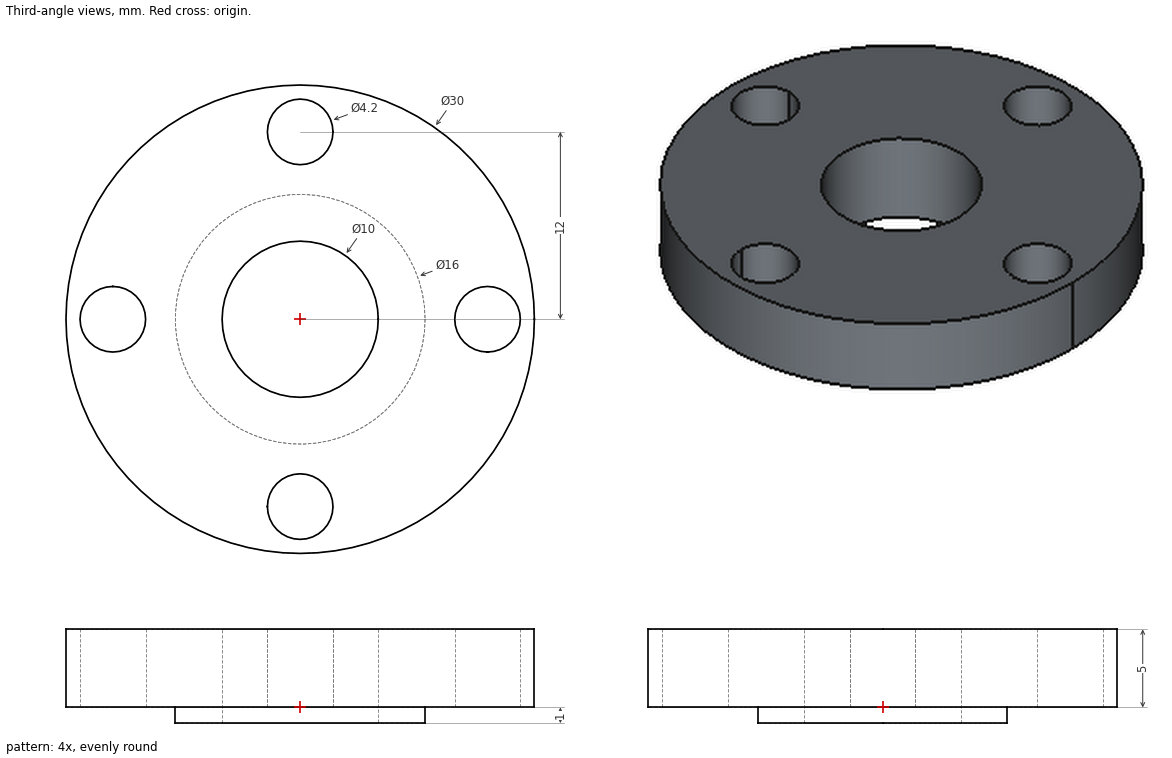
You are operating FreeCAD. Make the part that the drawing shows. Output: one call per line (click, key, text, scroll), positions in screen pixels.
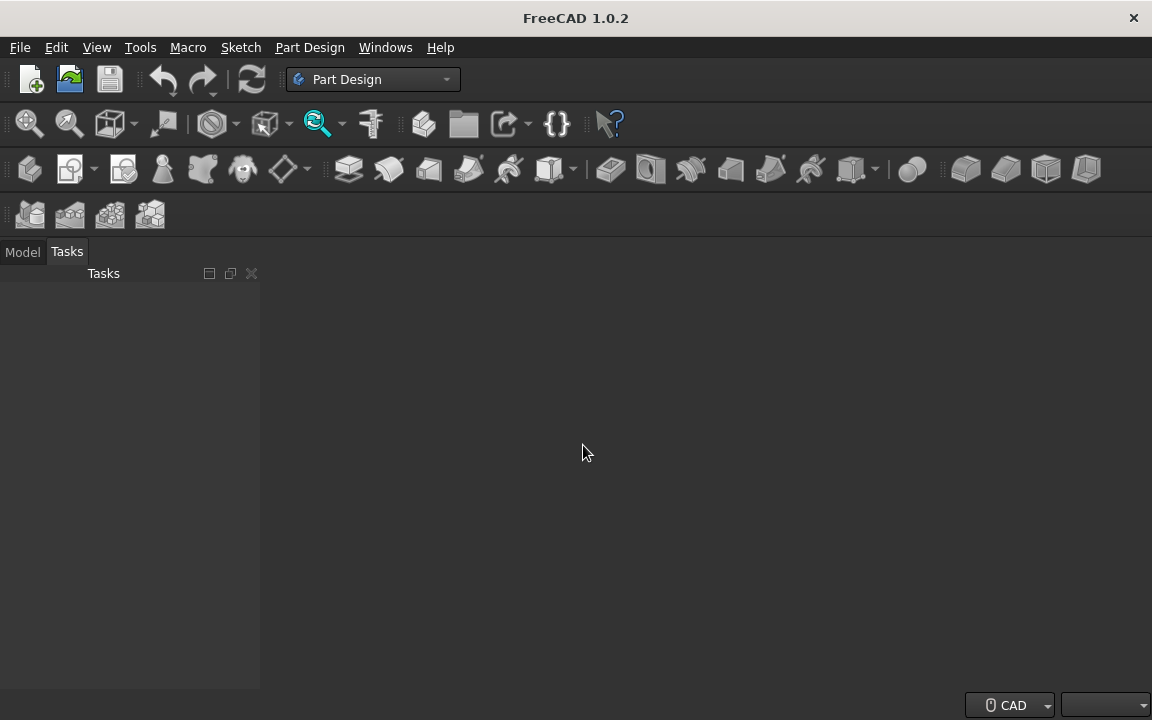
click(30, 80)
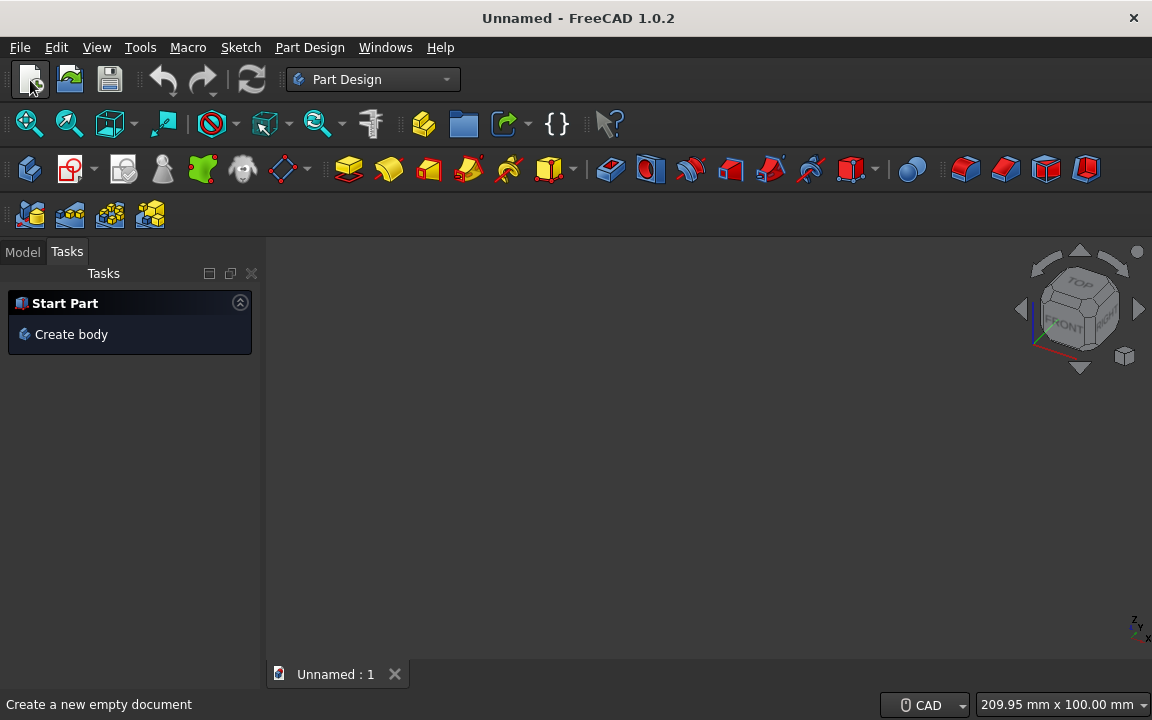
click(70, 170)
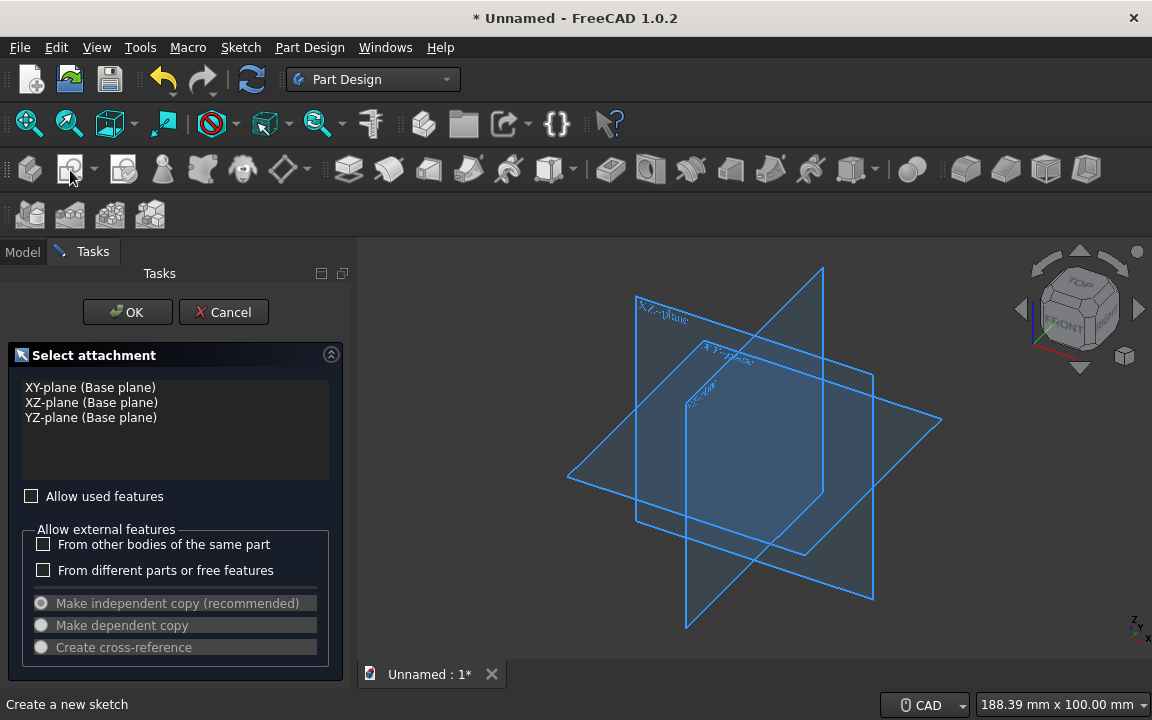
click(82, 388)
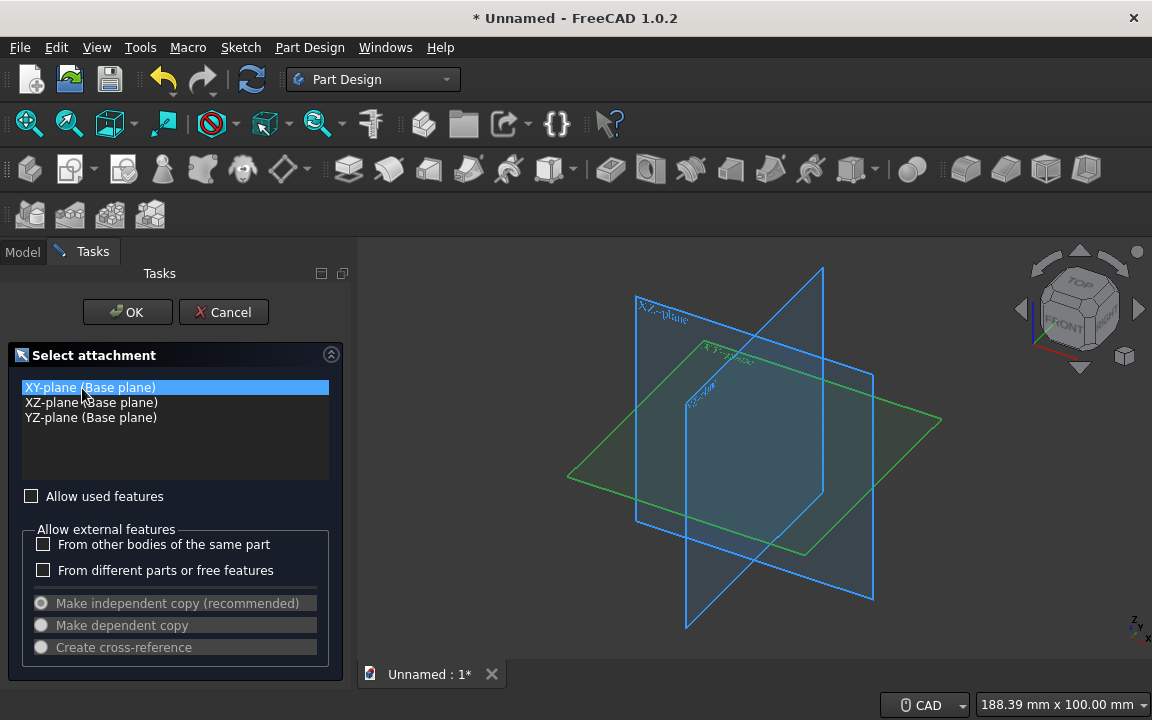
click(128, 312)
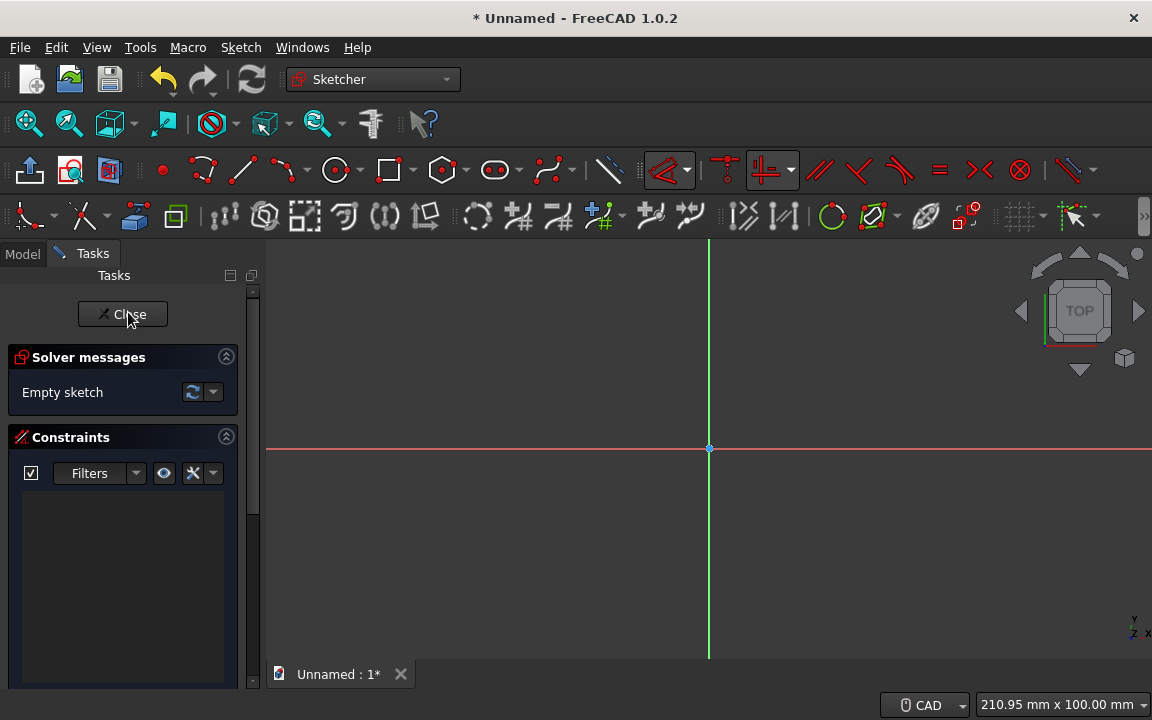
scroll(765, 449, up, 4)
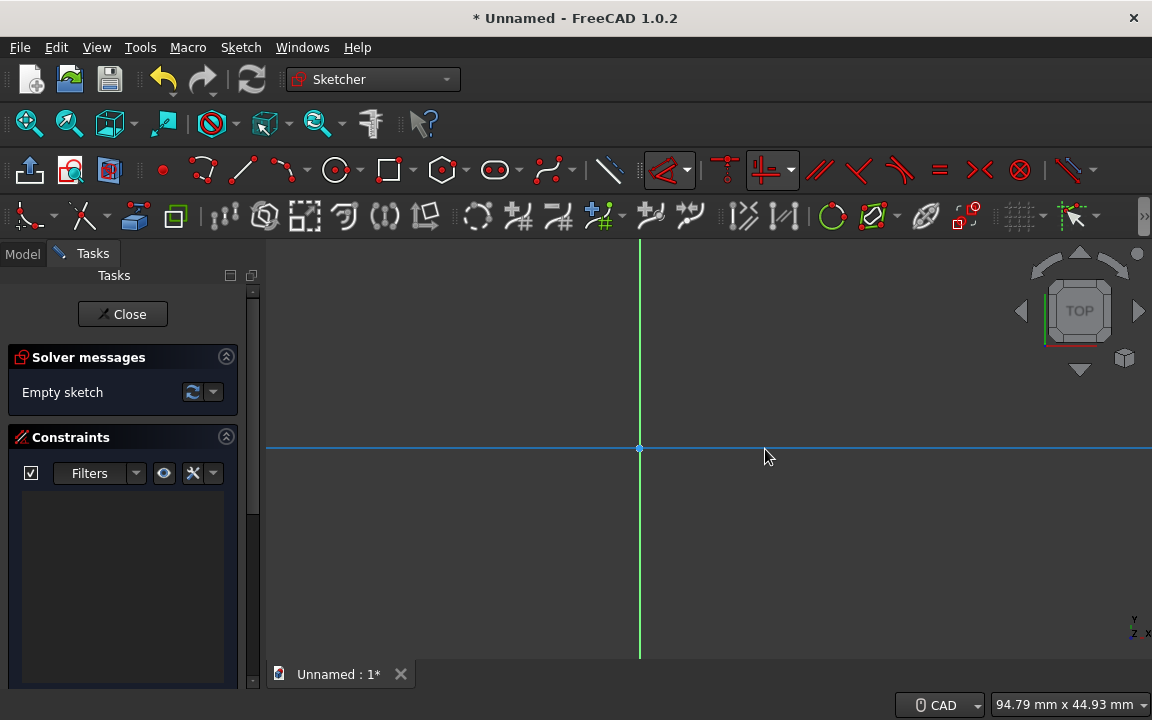
click(336, 170)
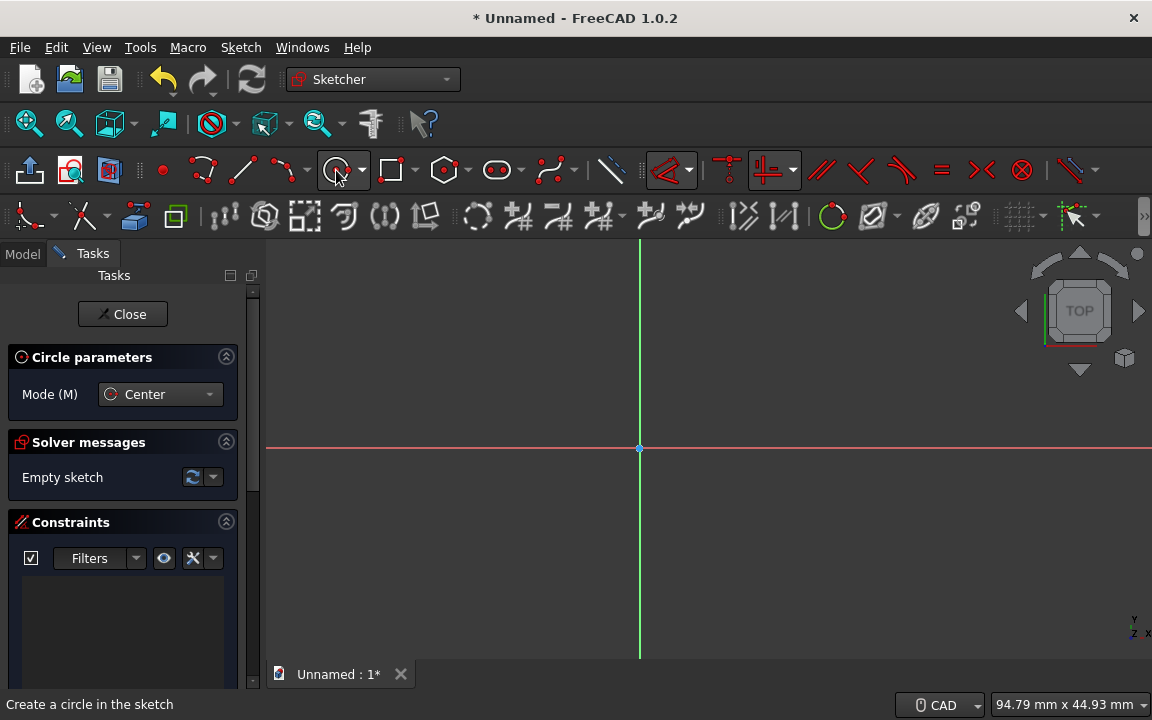
click(640, 448)
click(739, 349)
key(Escape)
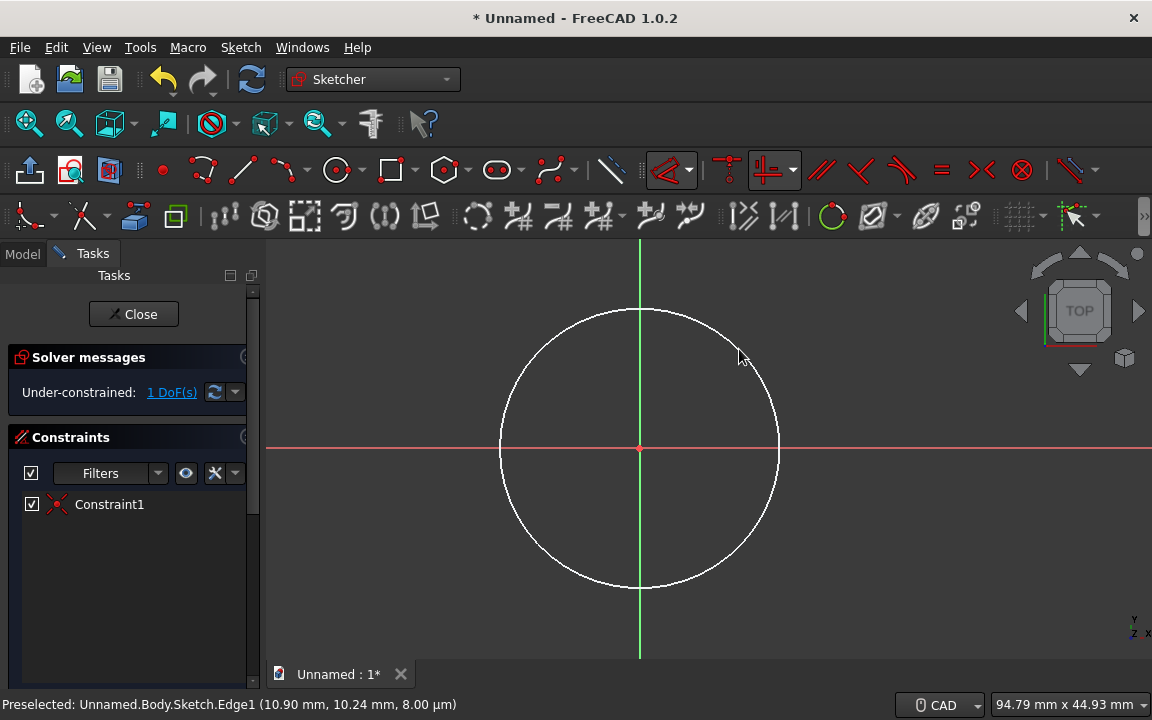
click(738, 349)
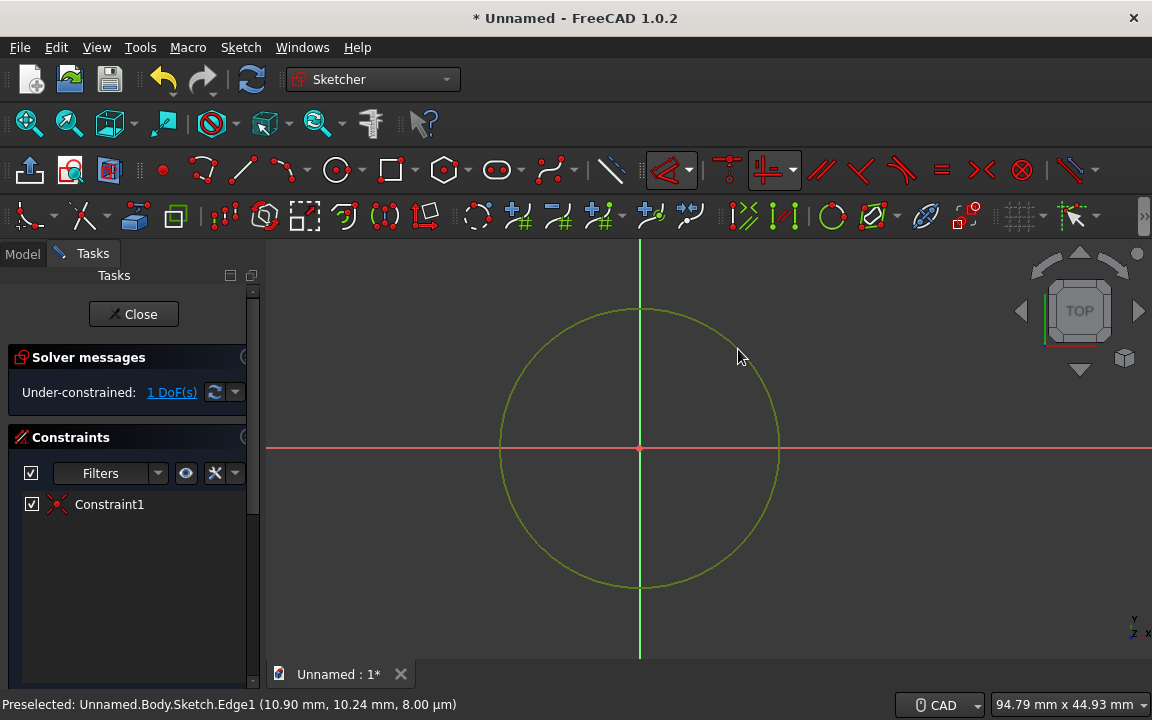
click(692, 170)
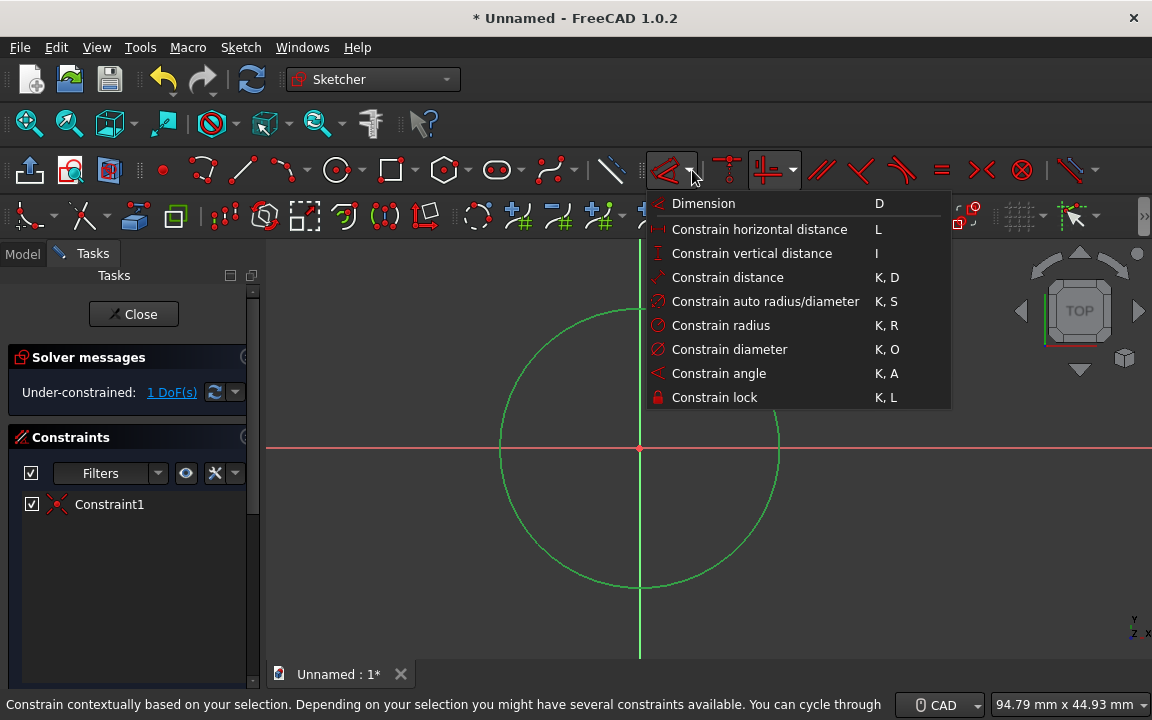
click(799, 349)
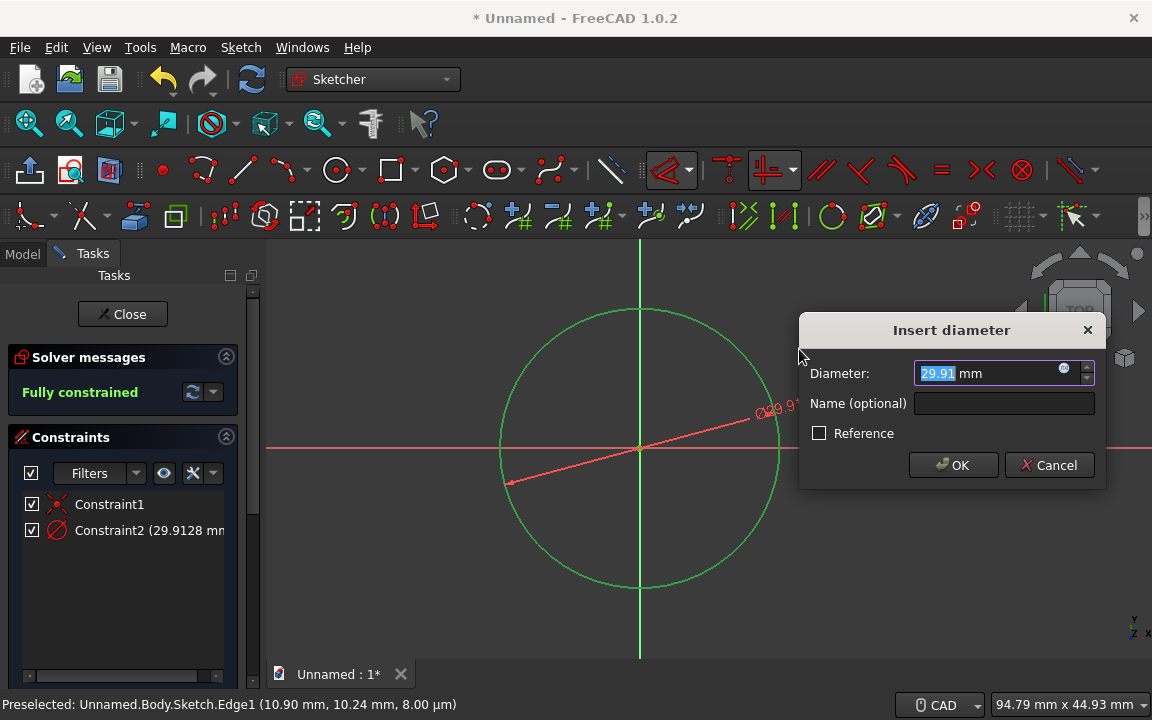
text(30)
key(Return)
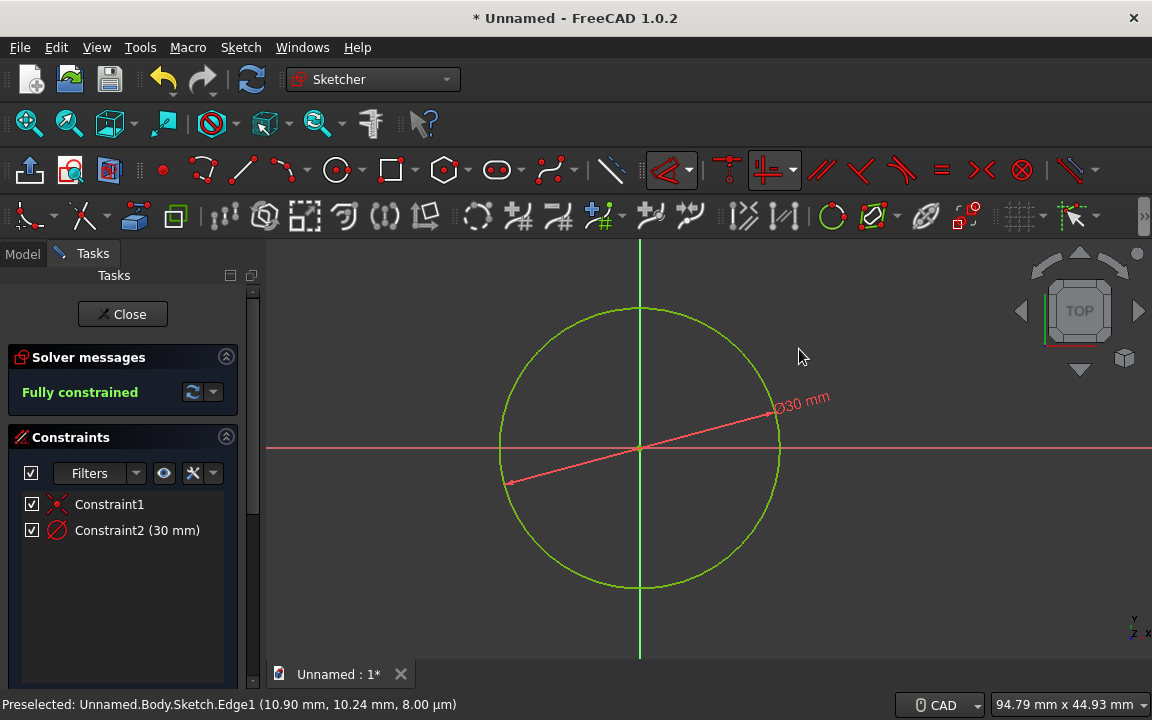
click(123, 314)